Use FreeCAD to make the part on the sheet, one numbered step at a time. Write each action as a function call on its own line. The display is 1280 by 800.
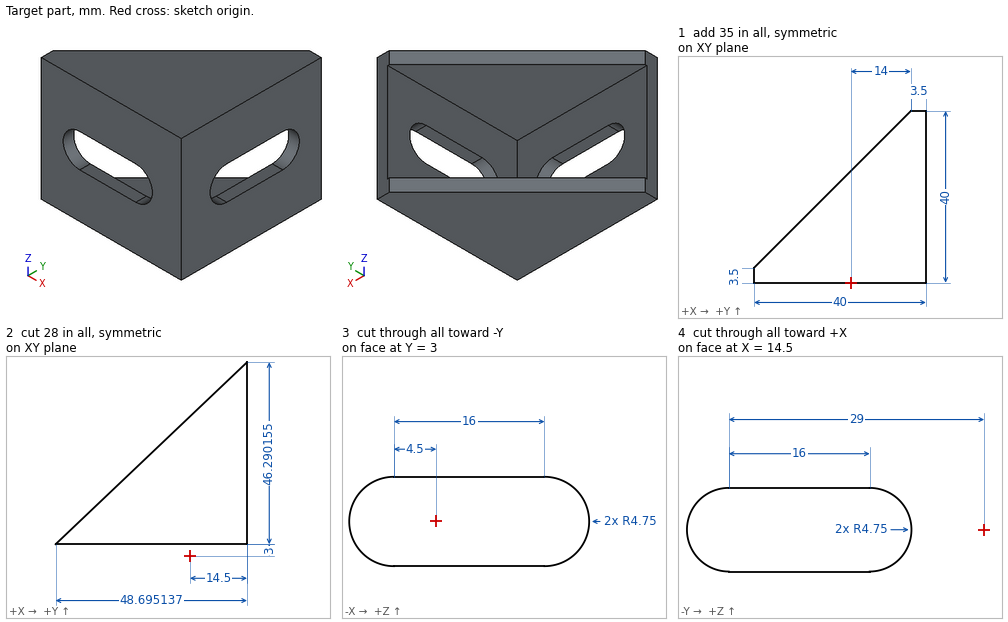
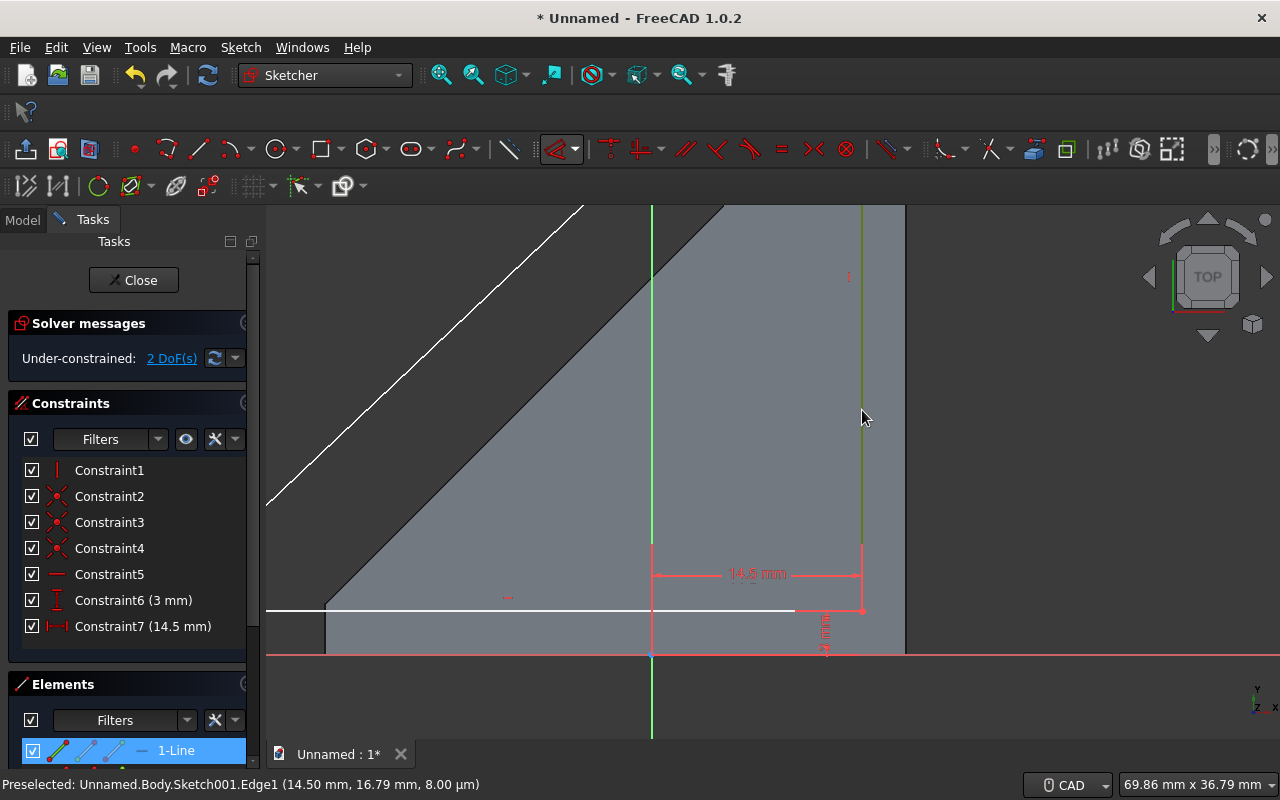
click(578, 150)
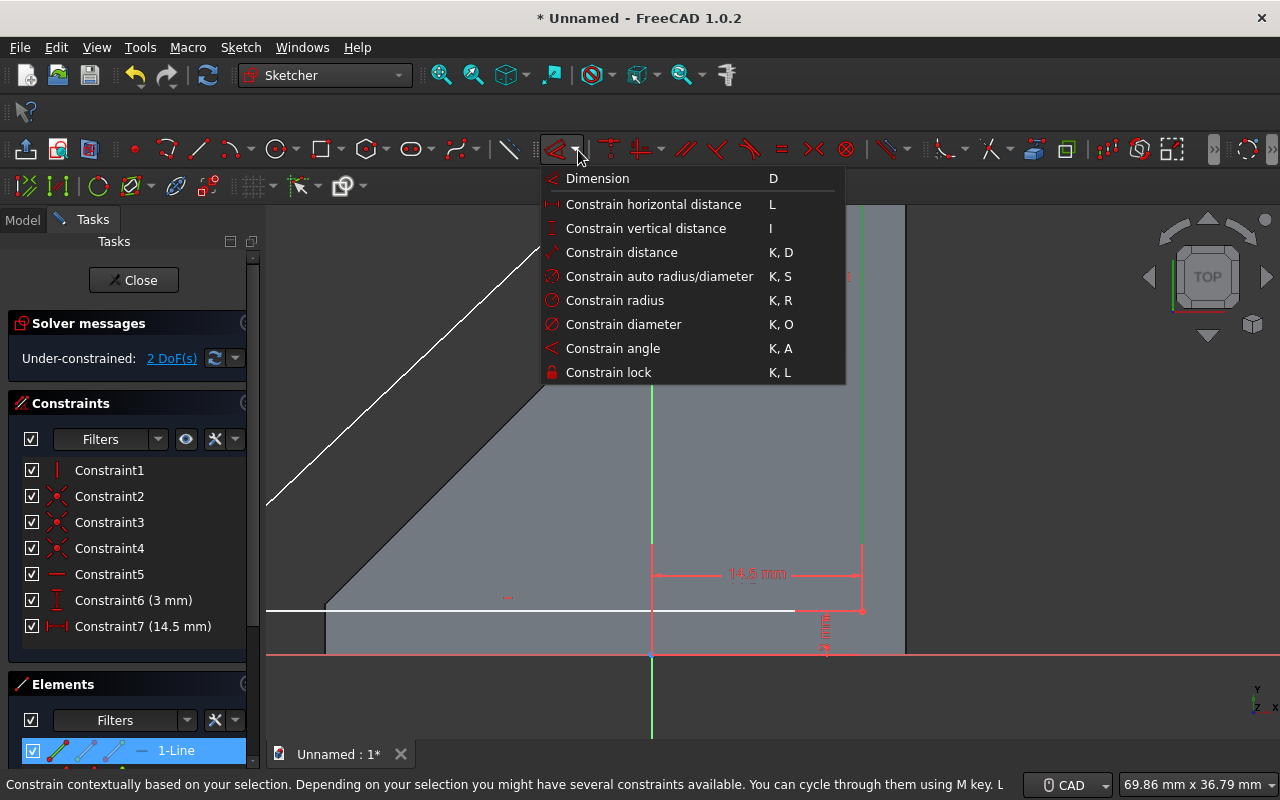
click(693, 228)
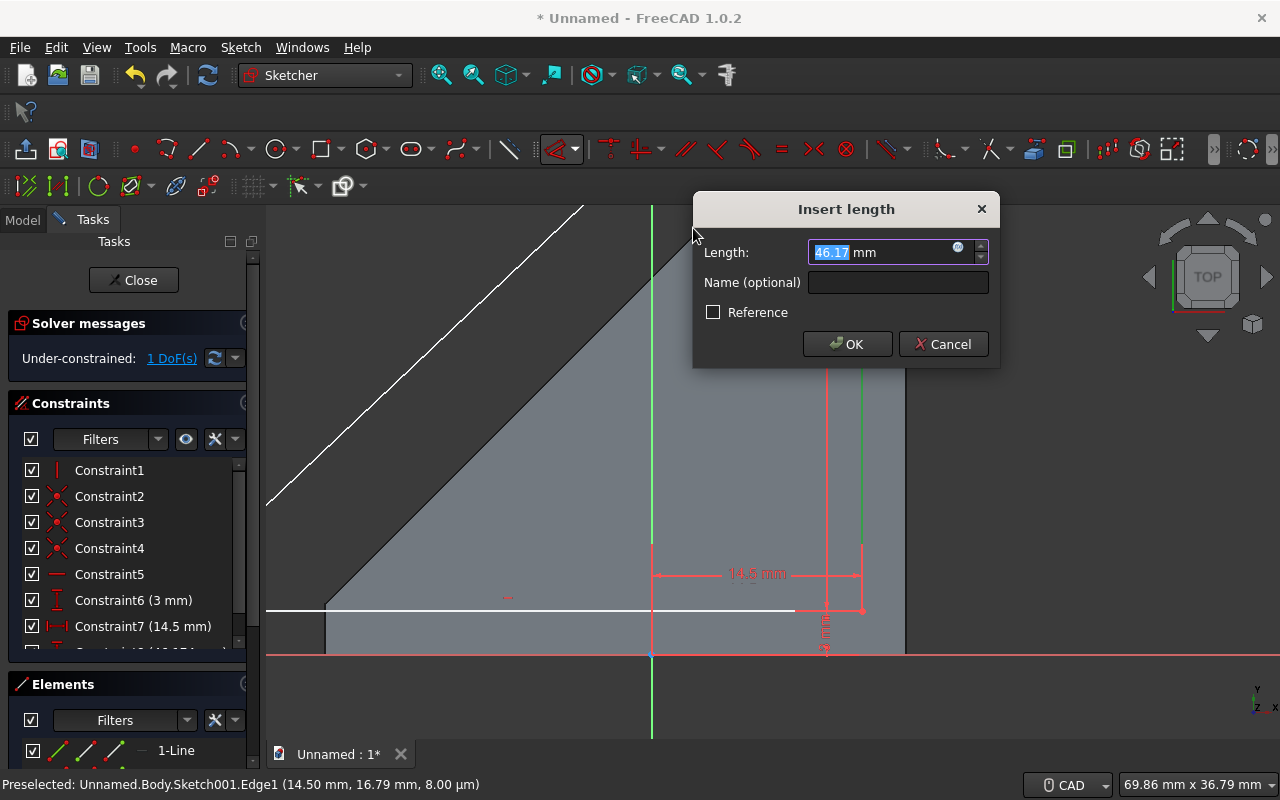
text(46.290155)
key(Return)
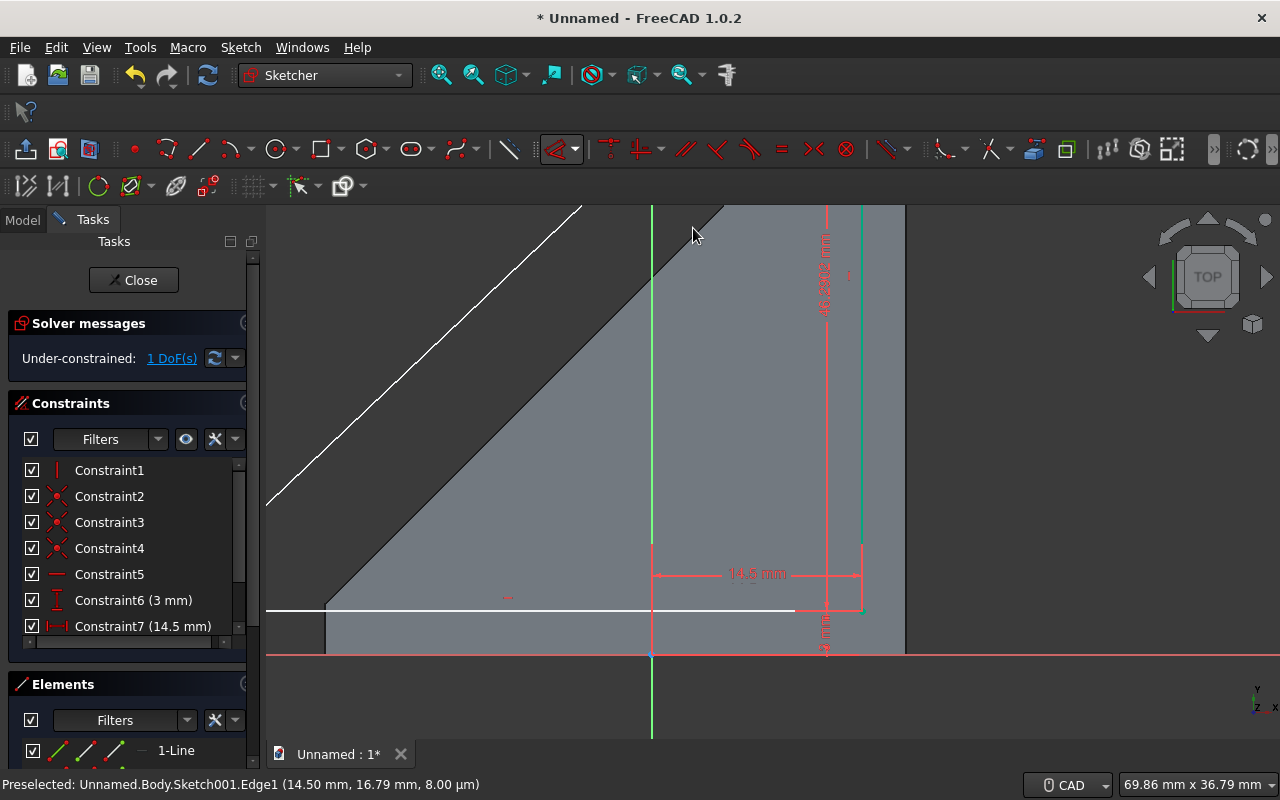
click(367, 611)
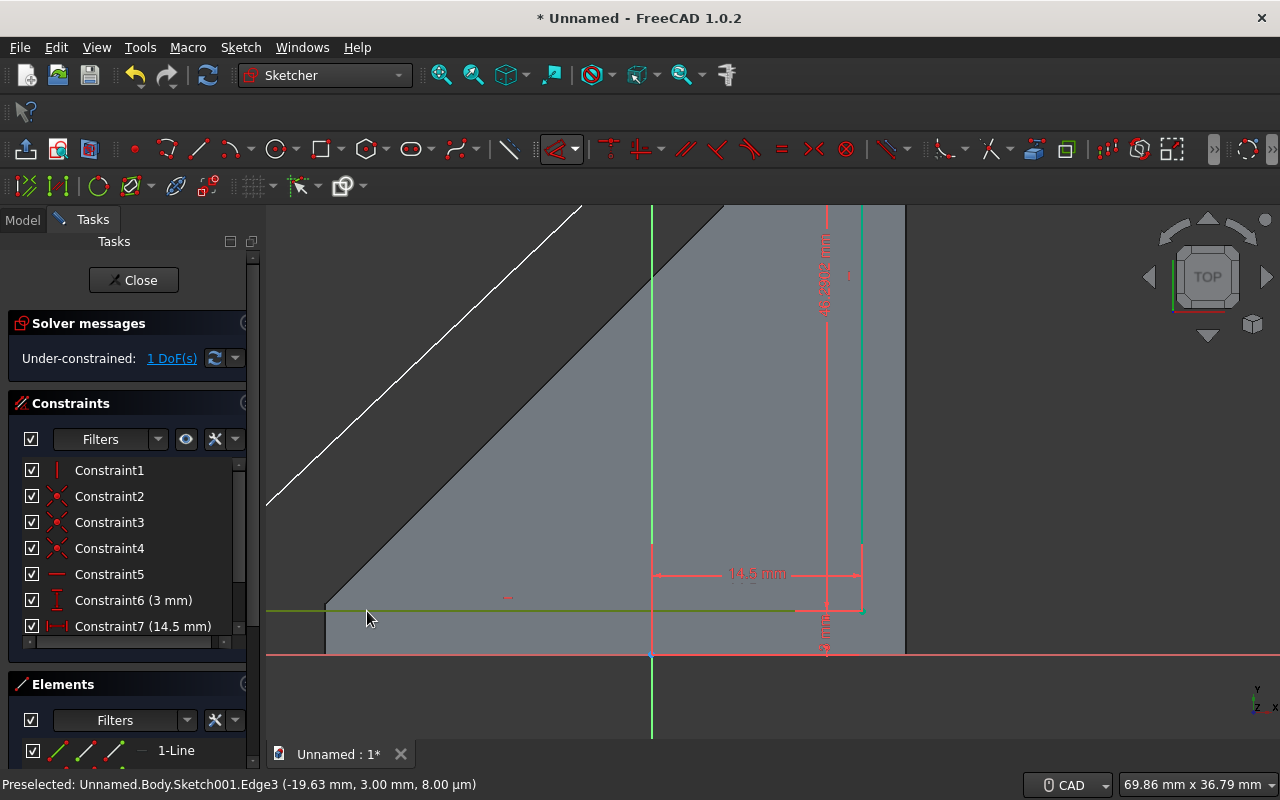
key(l)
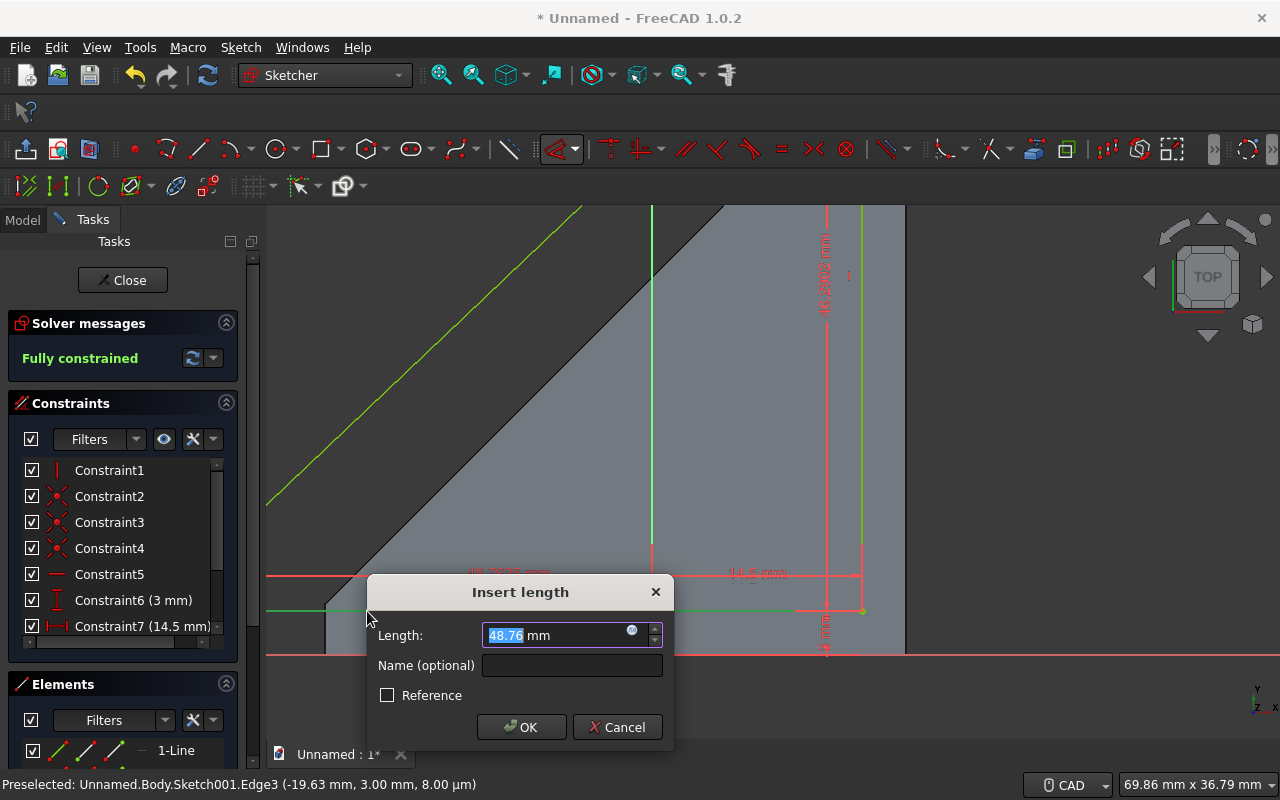
text(48.695137)
key(Return)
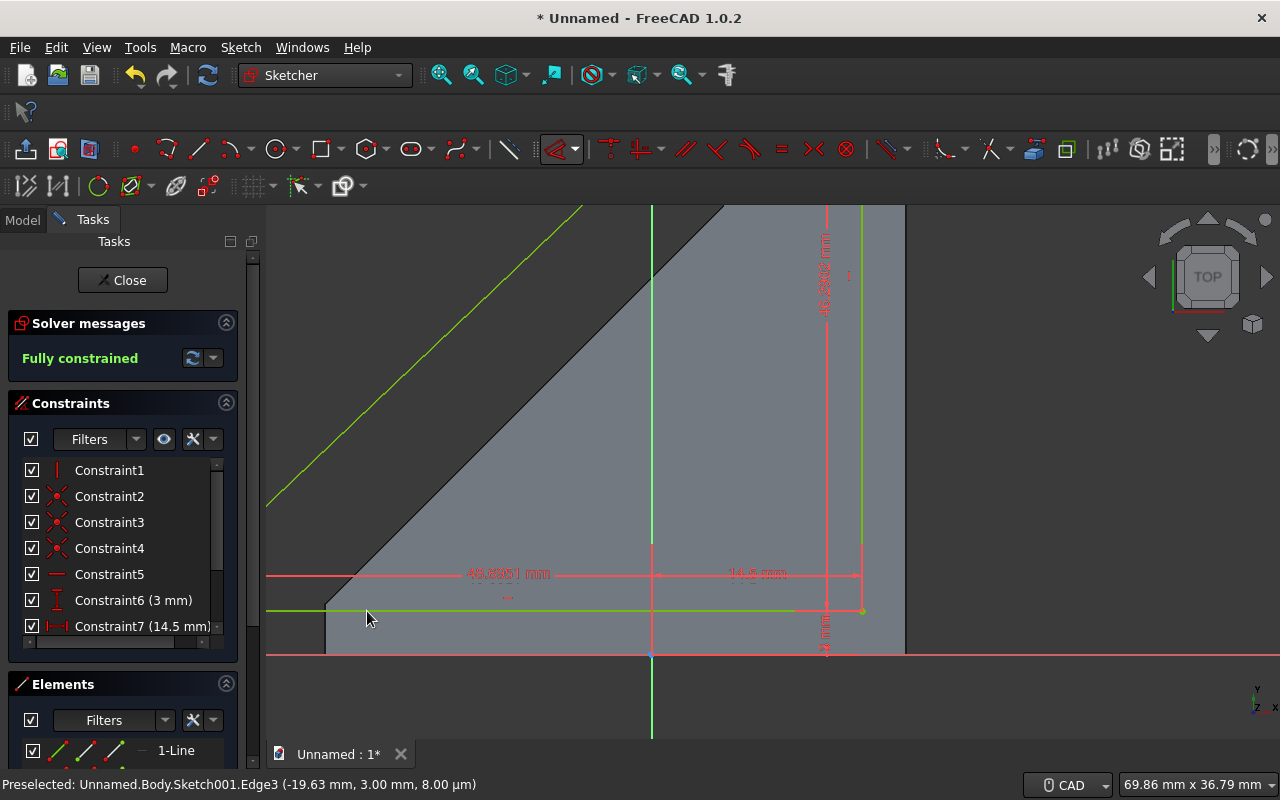
click(123, 280)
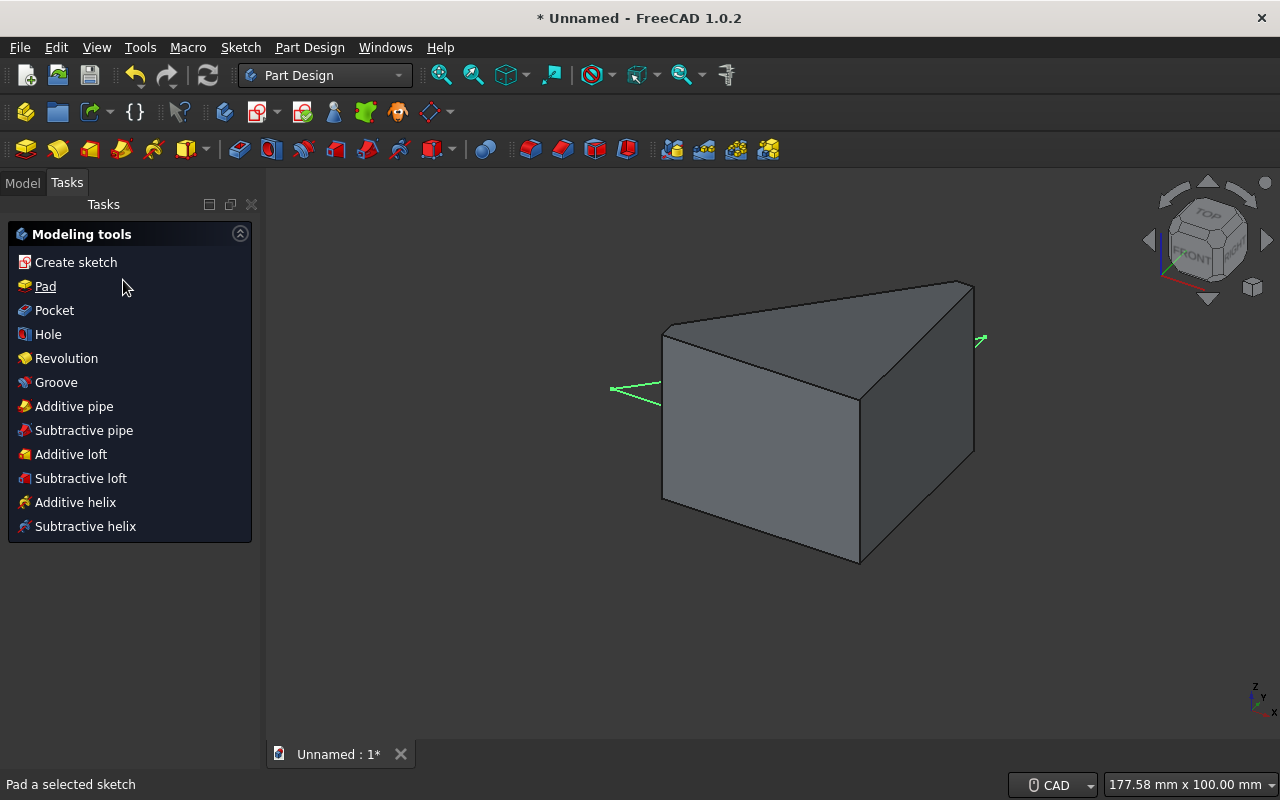
click(240, 150)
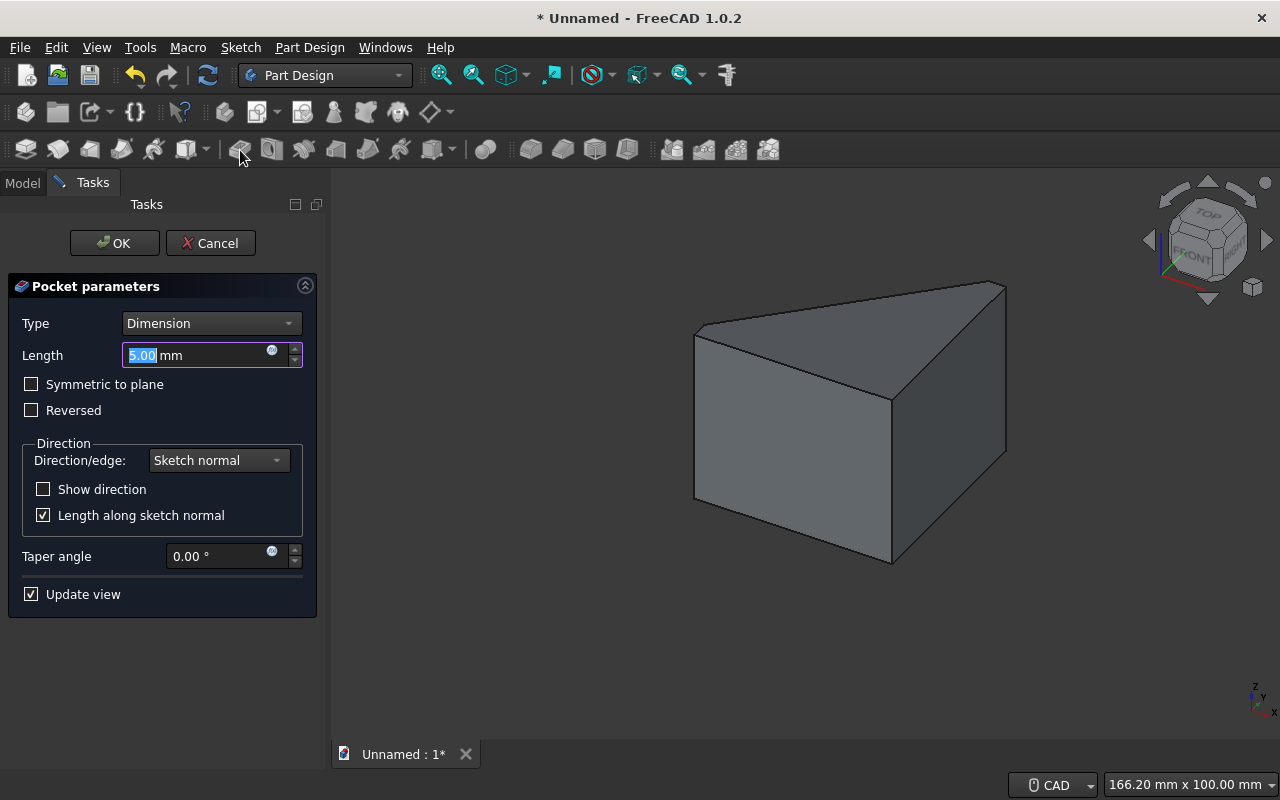
text(28)
key(Tab)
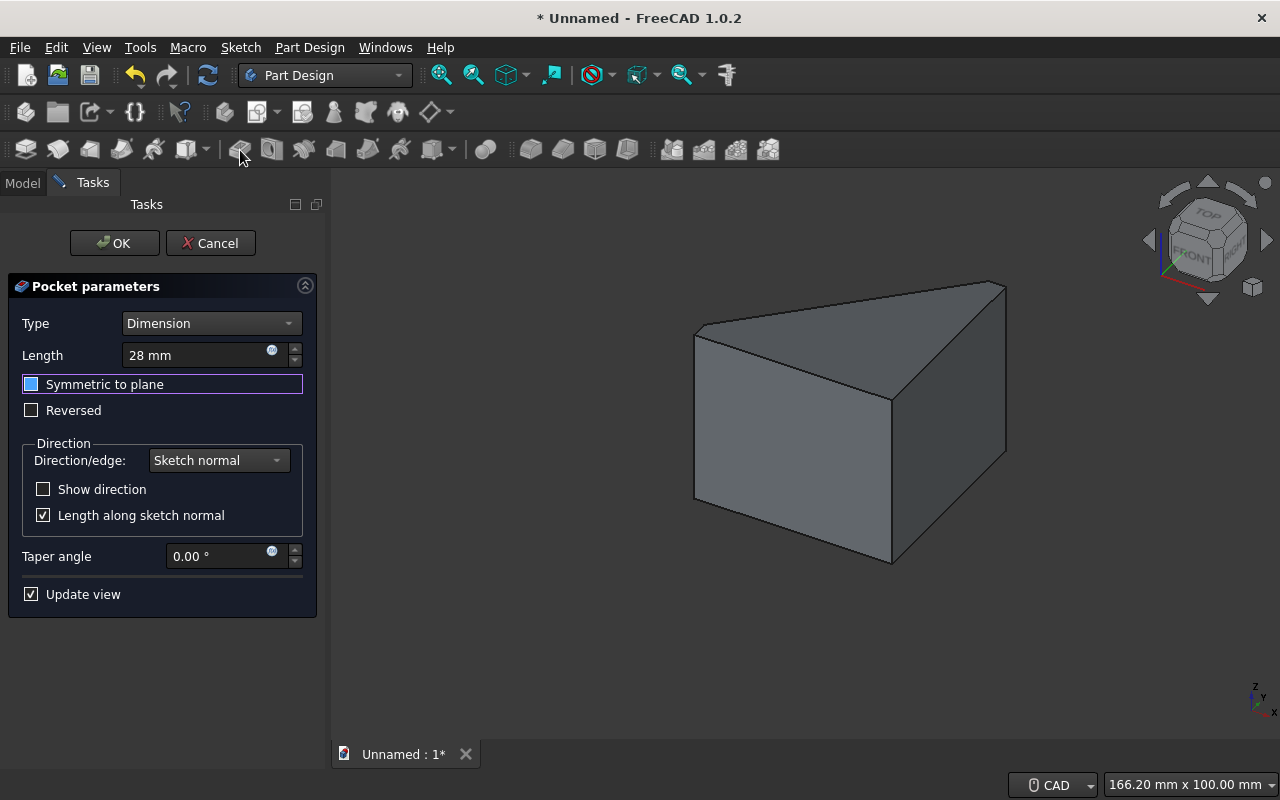
click(30, 384)